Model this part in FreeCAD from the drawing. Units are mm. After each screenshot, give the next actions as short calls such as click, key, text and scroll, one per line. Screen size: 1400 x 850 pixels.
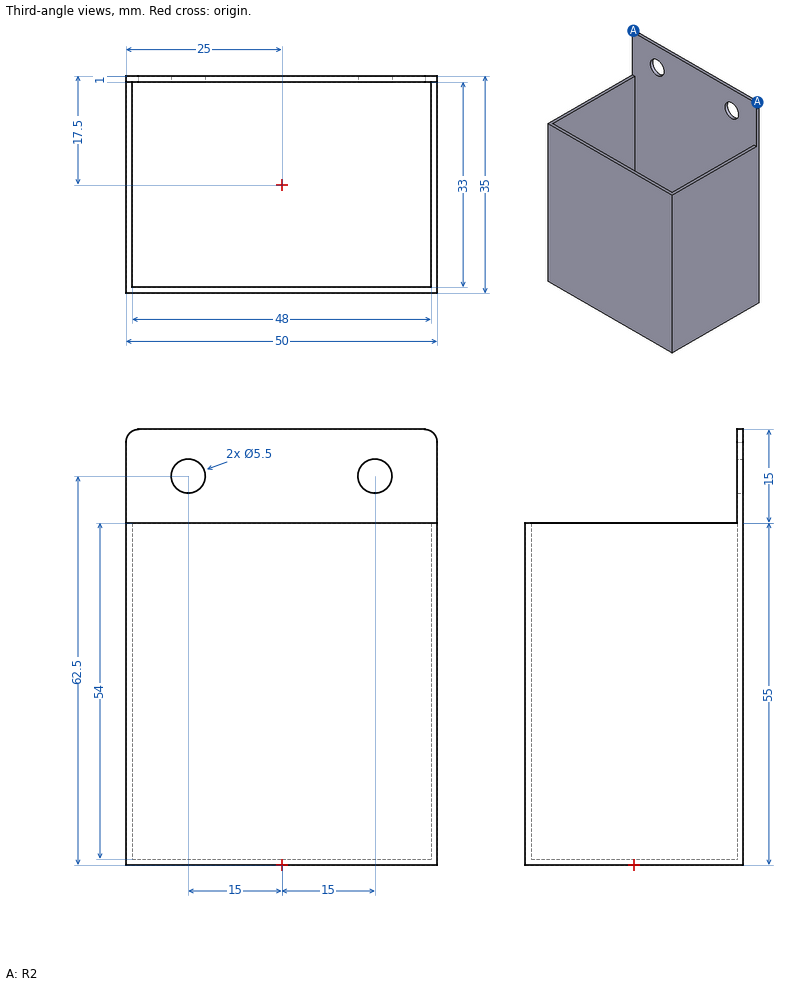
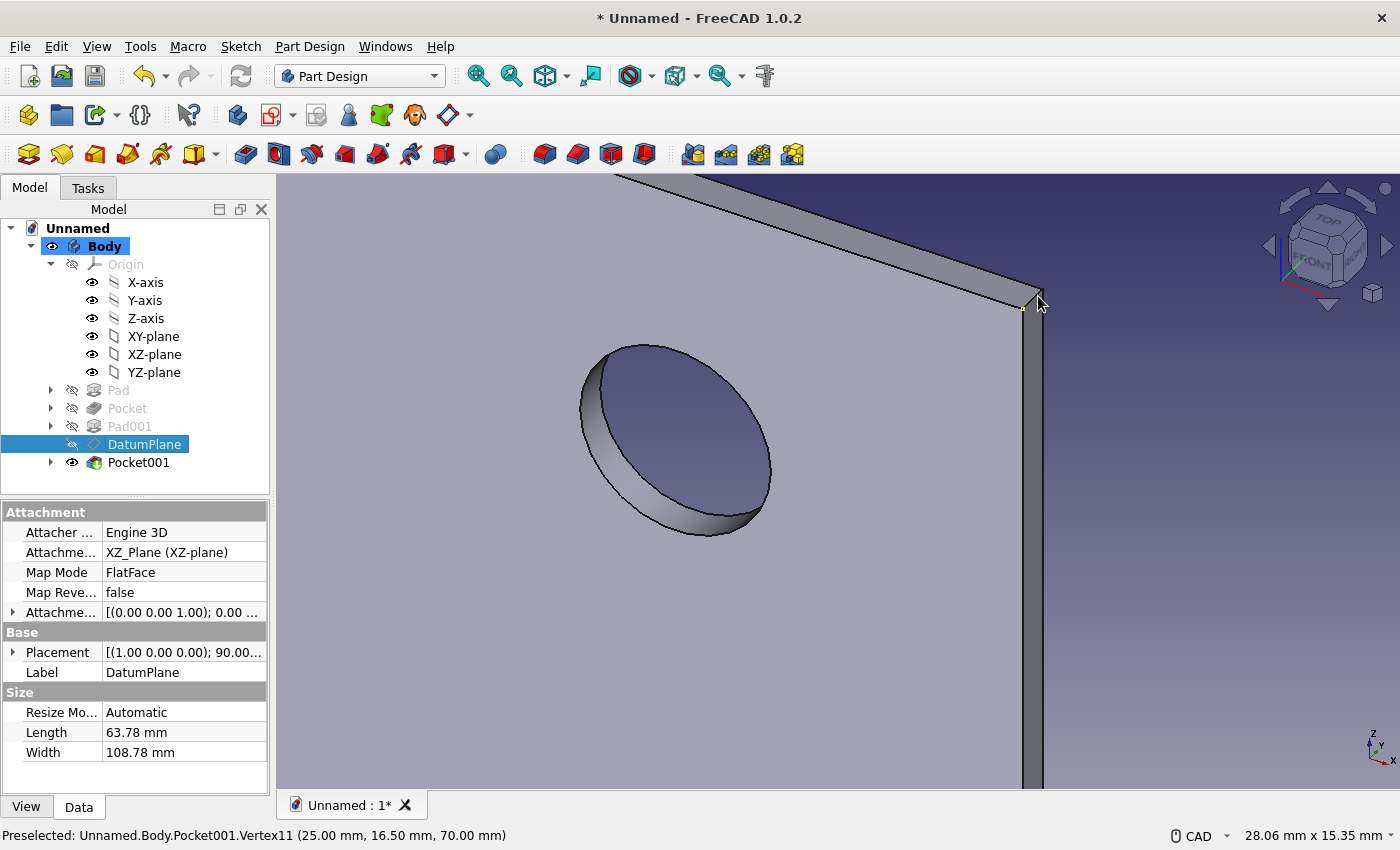
click(1033, 298)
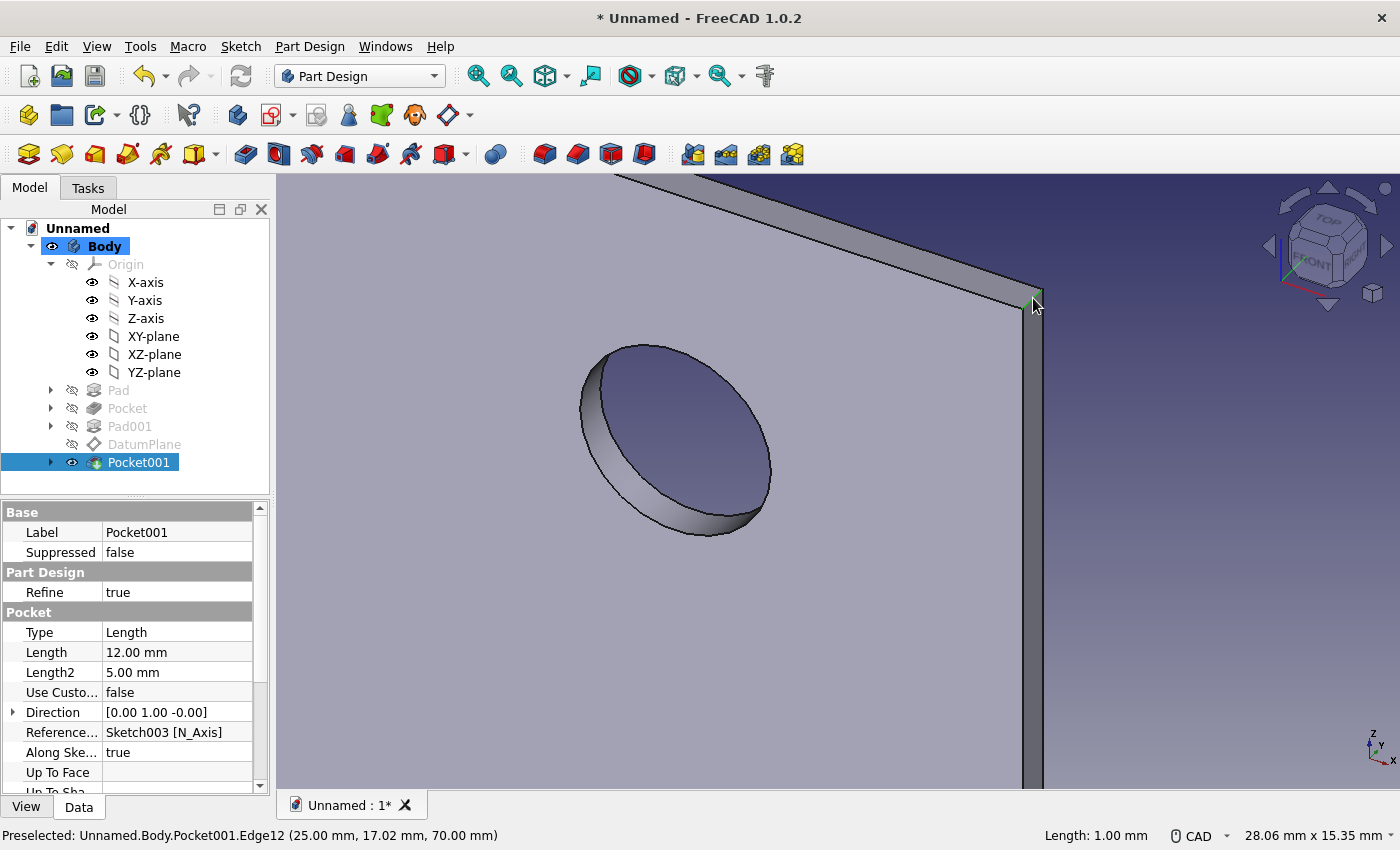
click(479, 76)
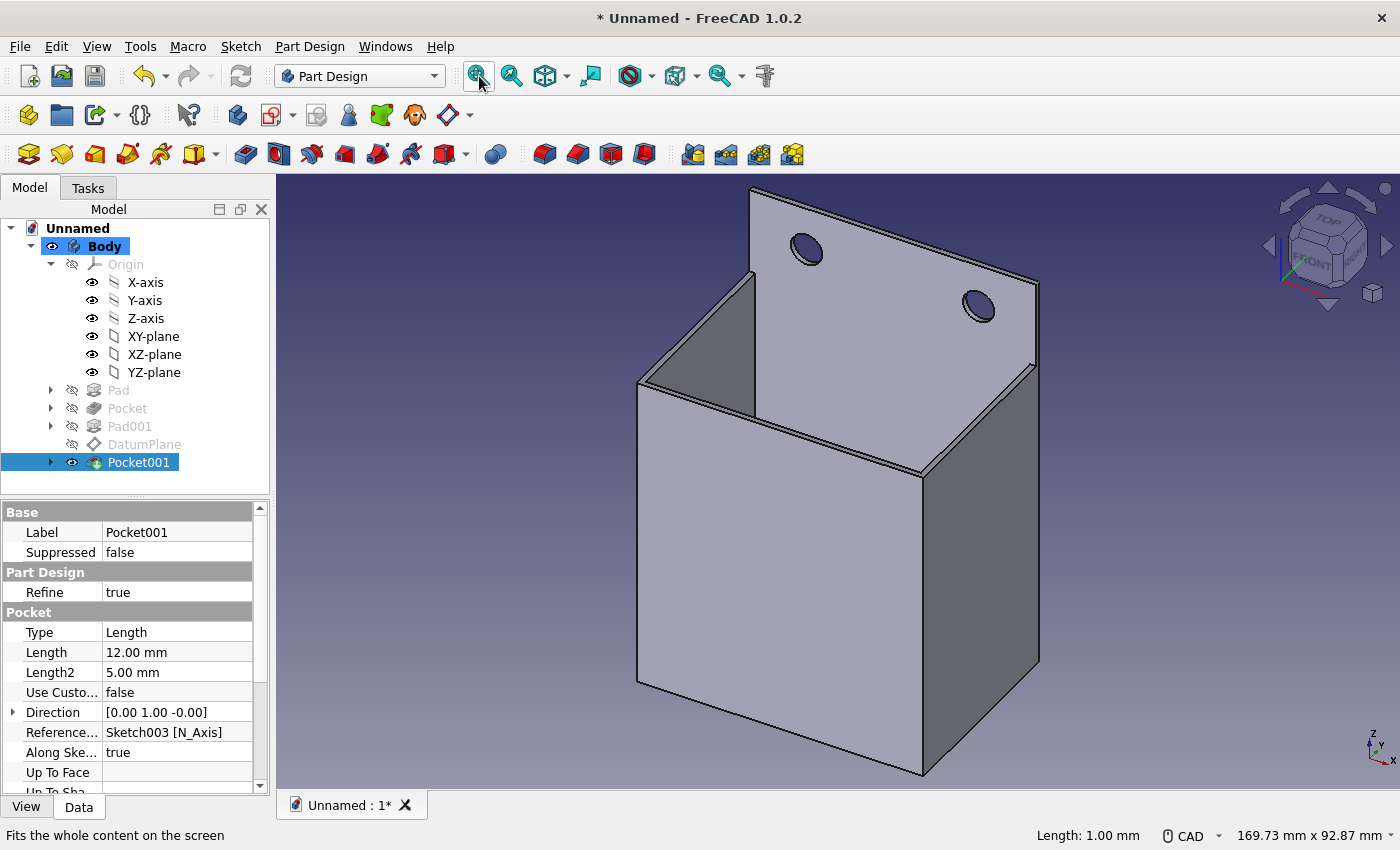
key(0)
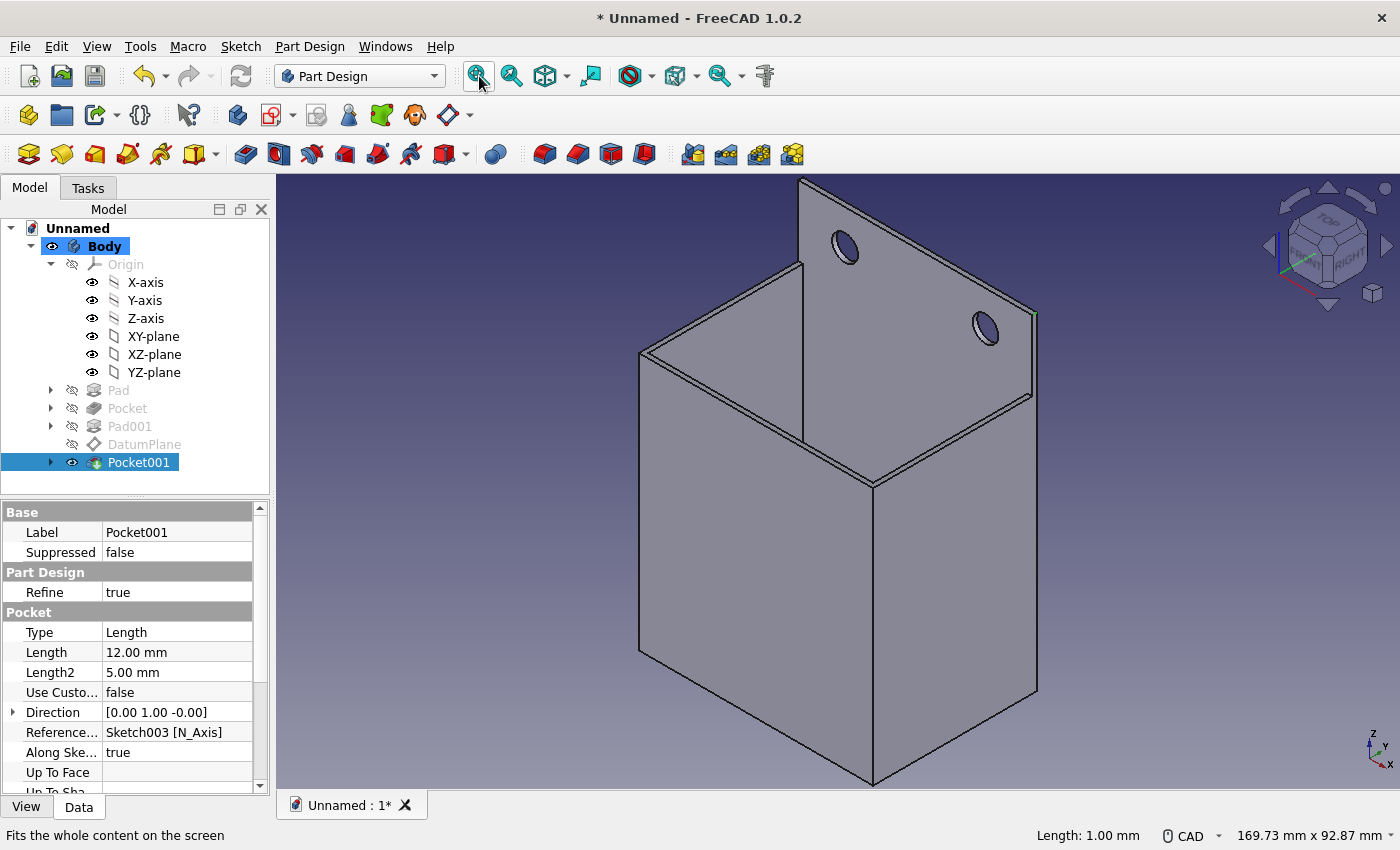
key(2)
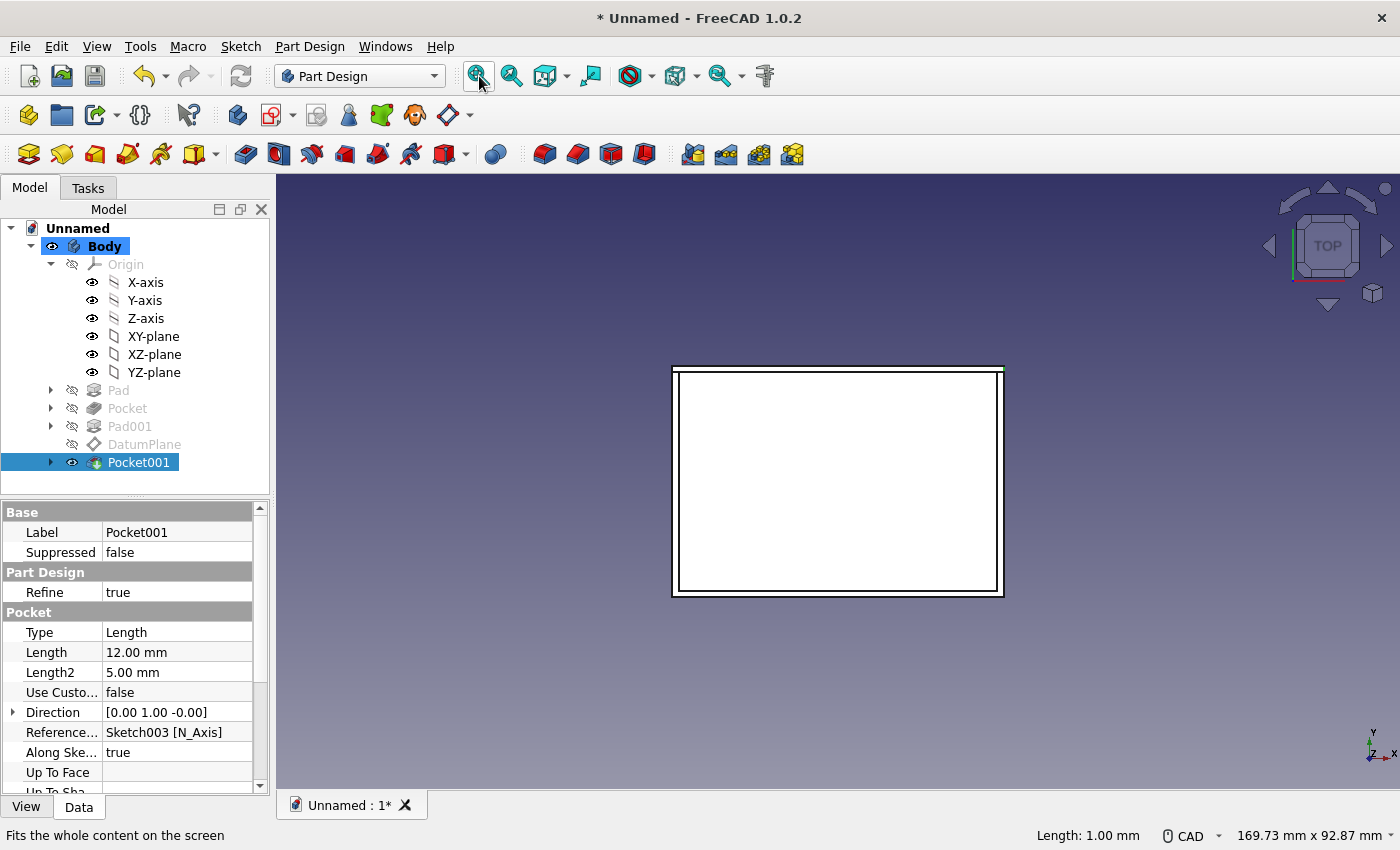
click(479, 76)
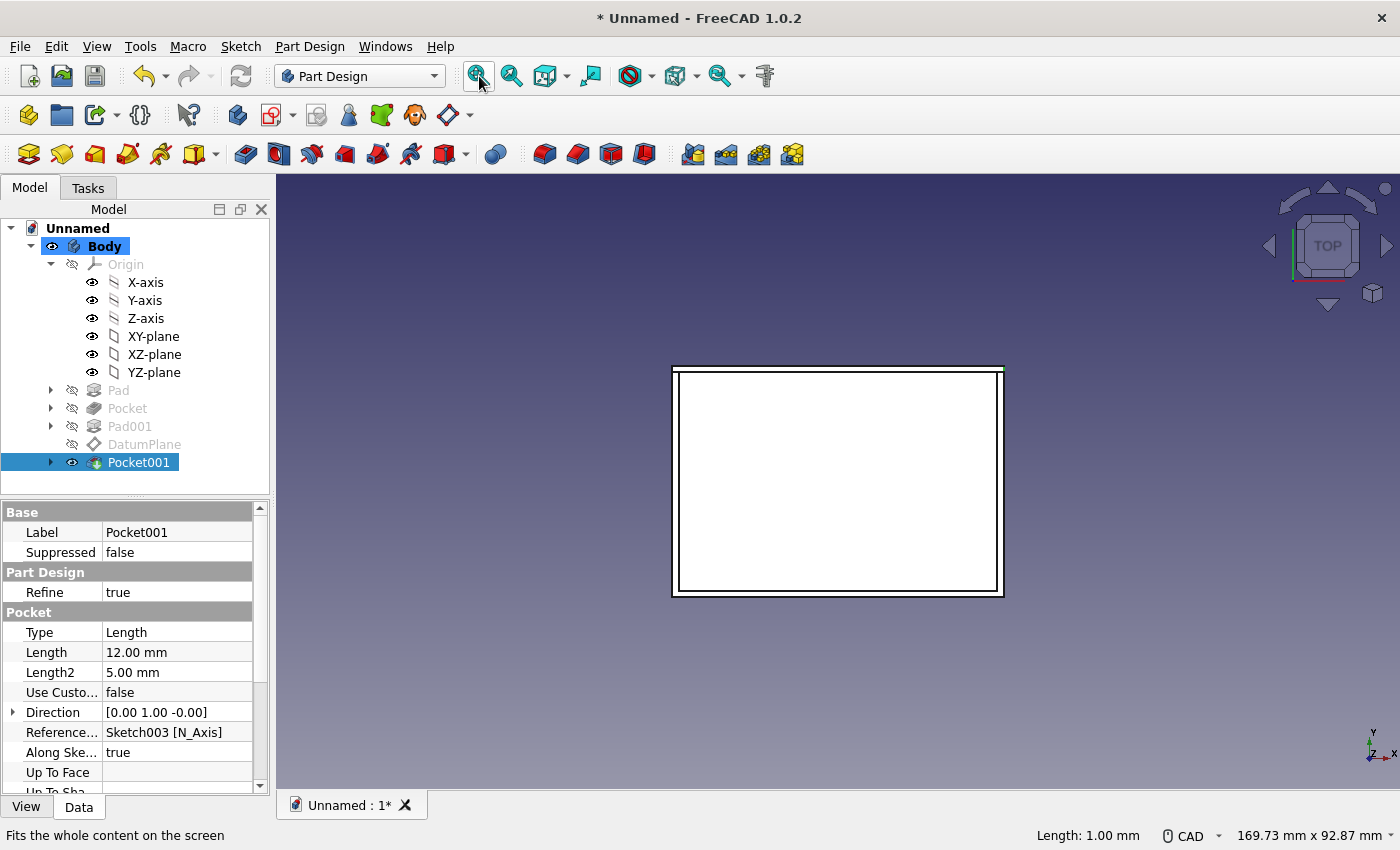
scroll(672, 368, up, 9)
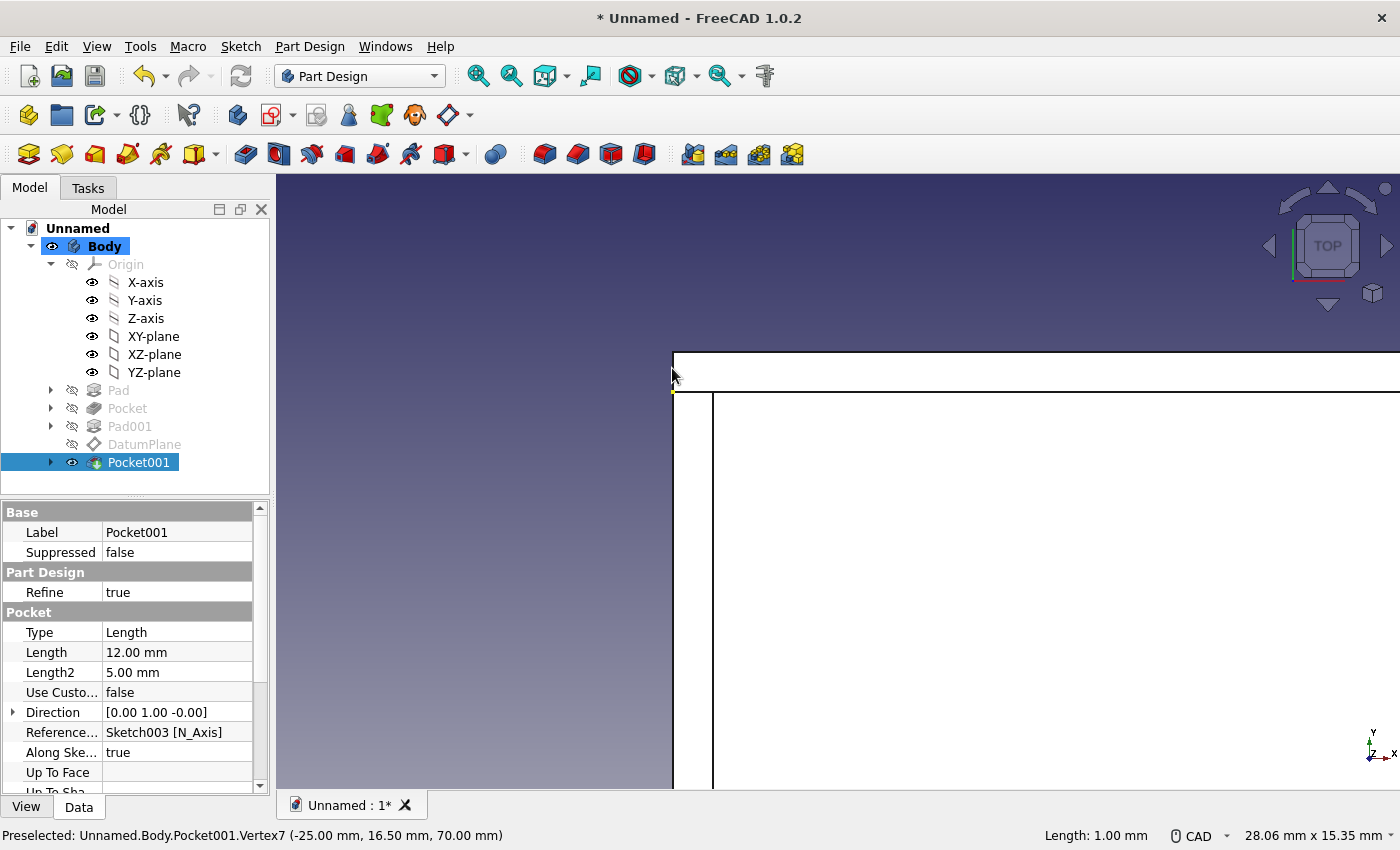
click(673, 371, ctrl)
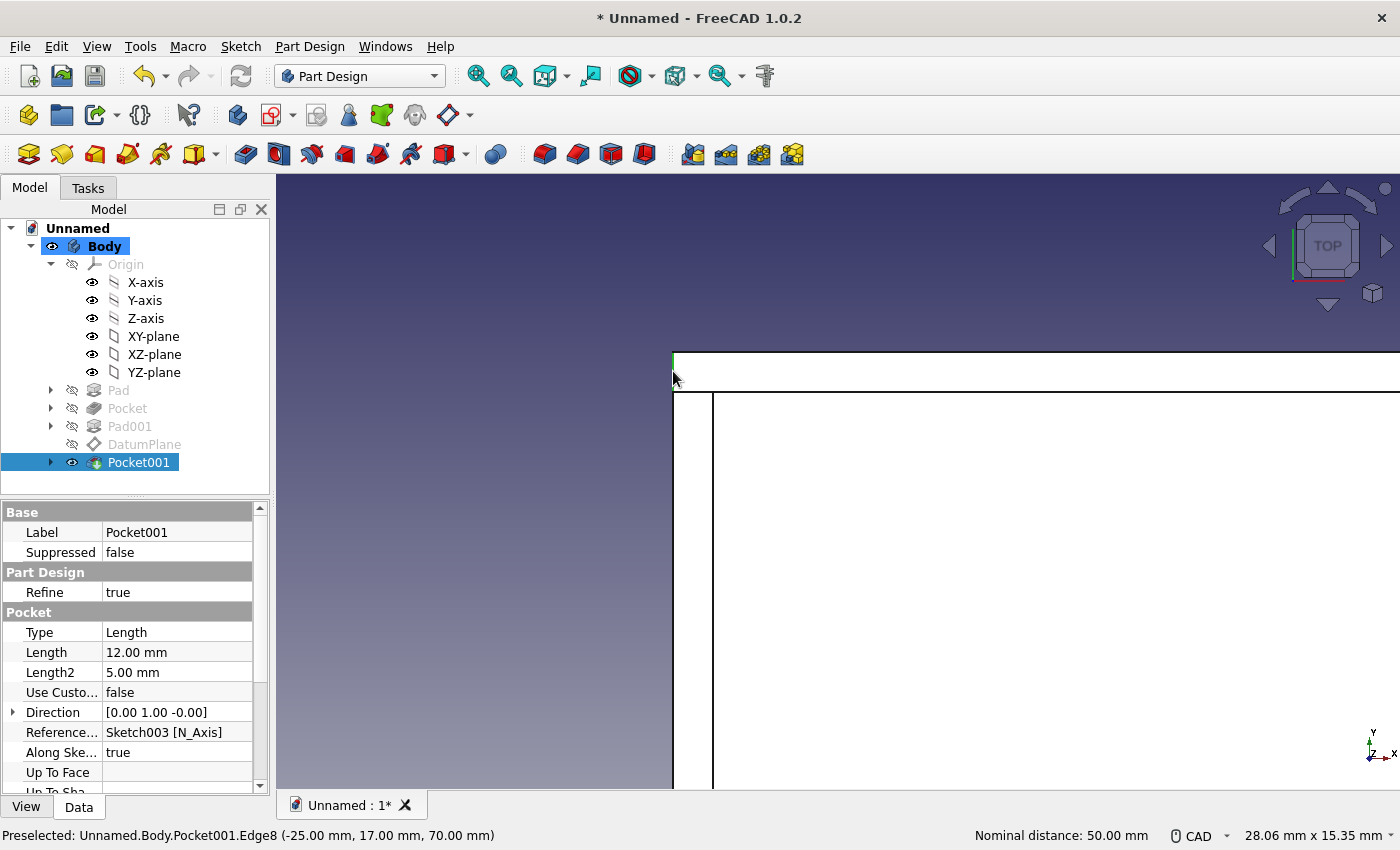
click(545, 154)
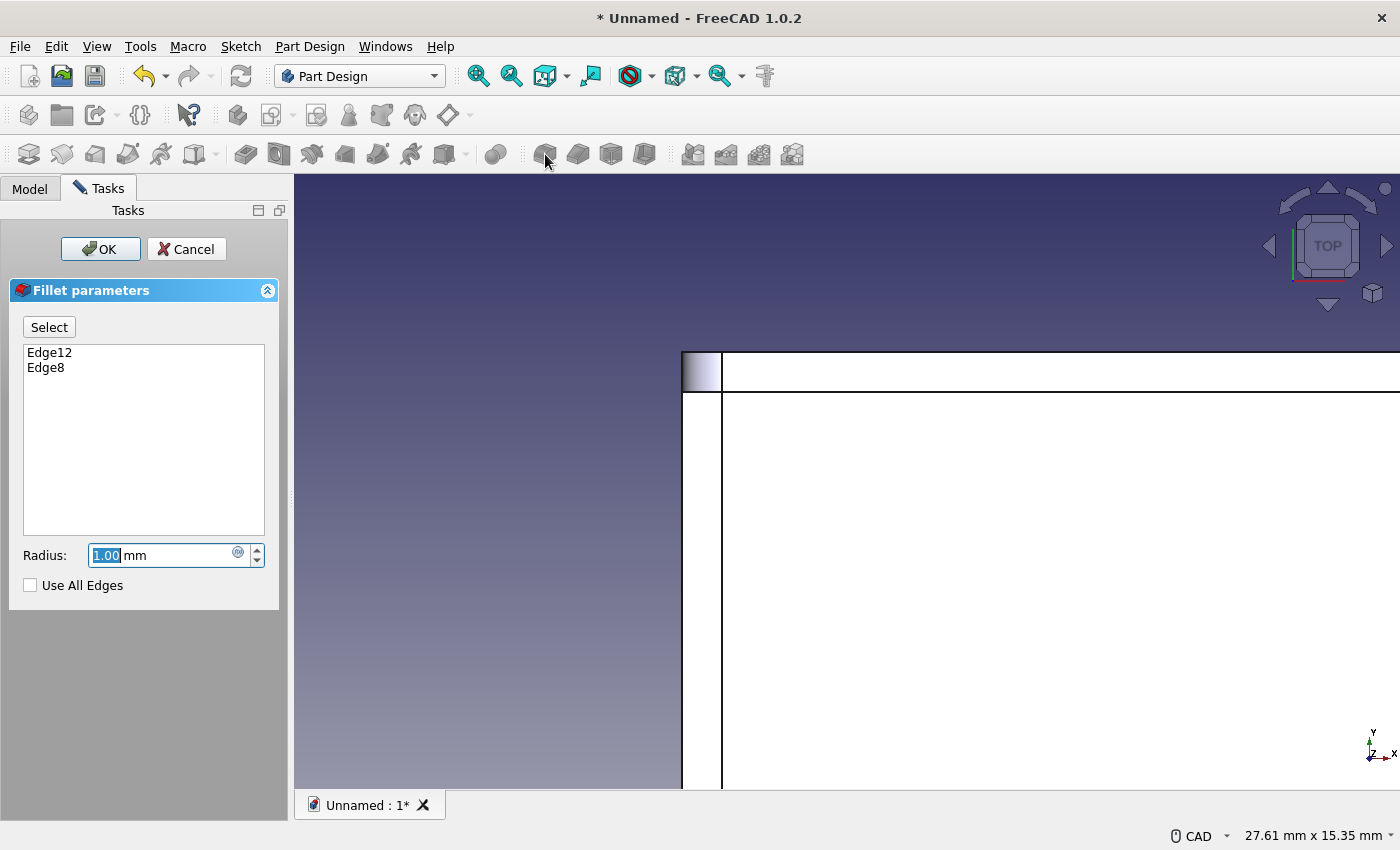
text(2)
key(Tab)